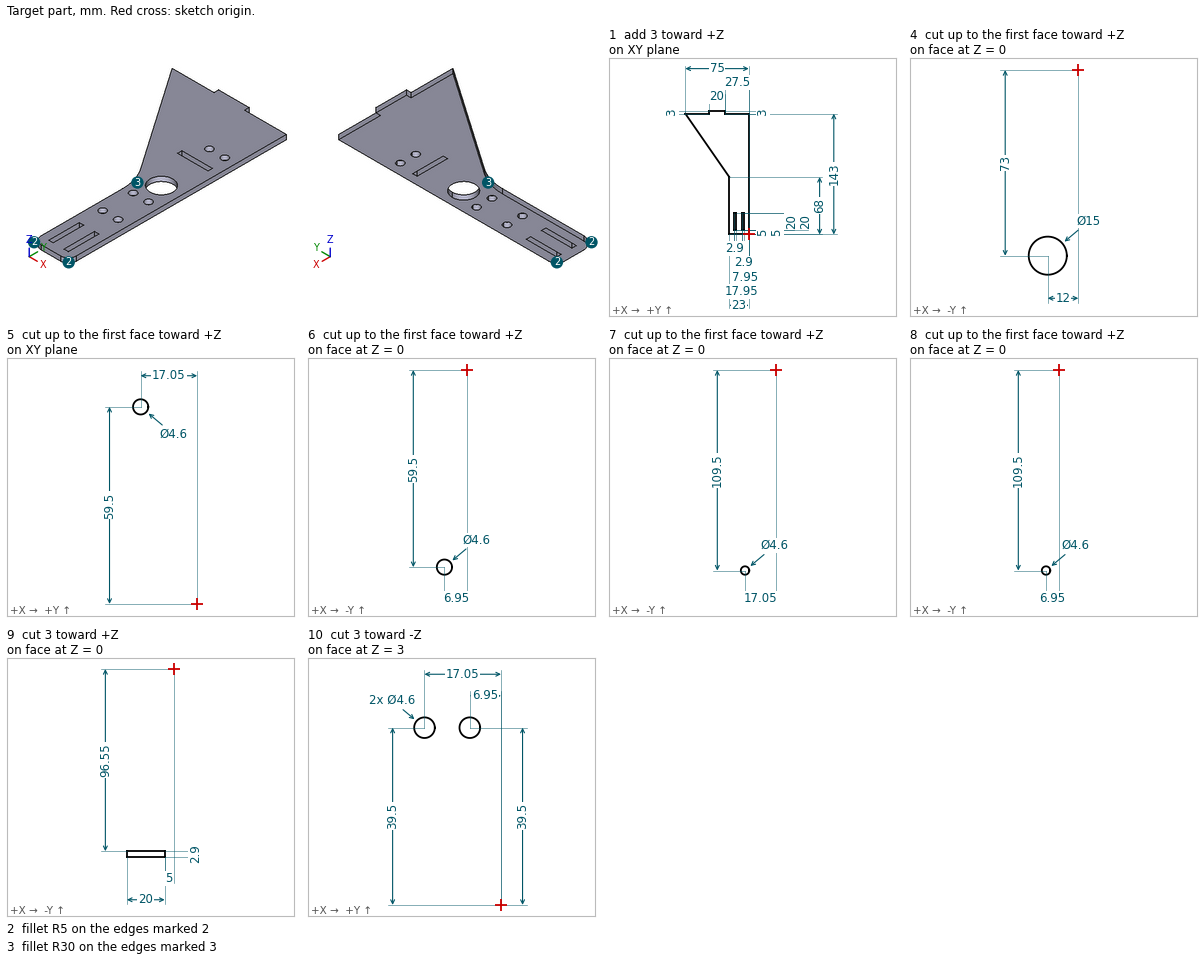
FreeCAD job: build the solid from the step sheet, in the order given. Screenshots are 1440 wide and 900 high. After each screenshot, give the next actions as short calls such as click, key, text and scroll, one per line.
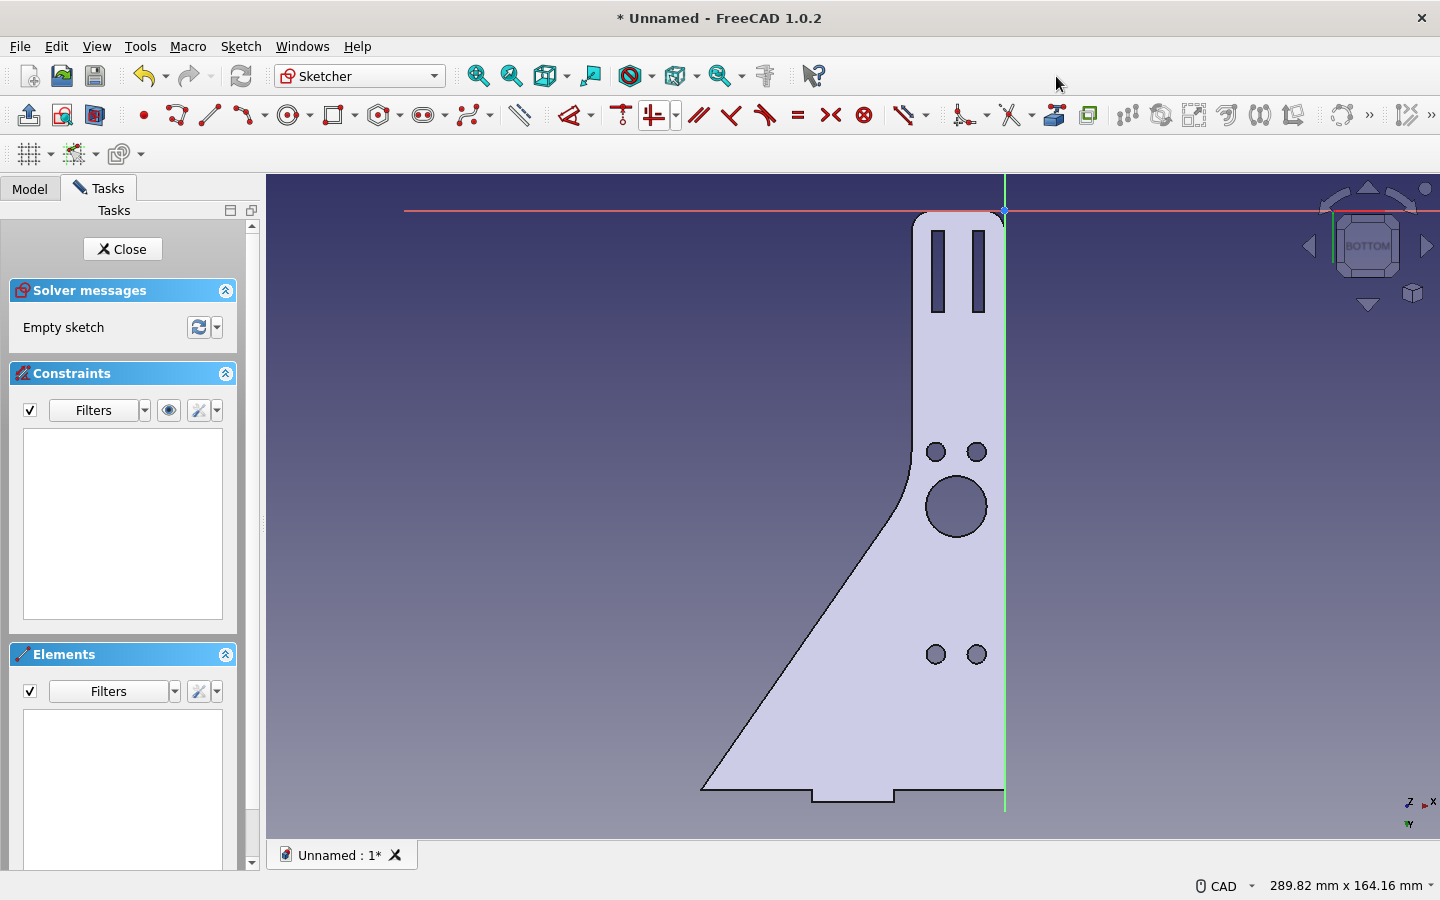
scroll(964, 620, up, 11)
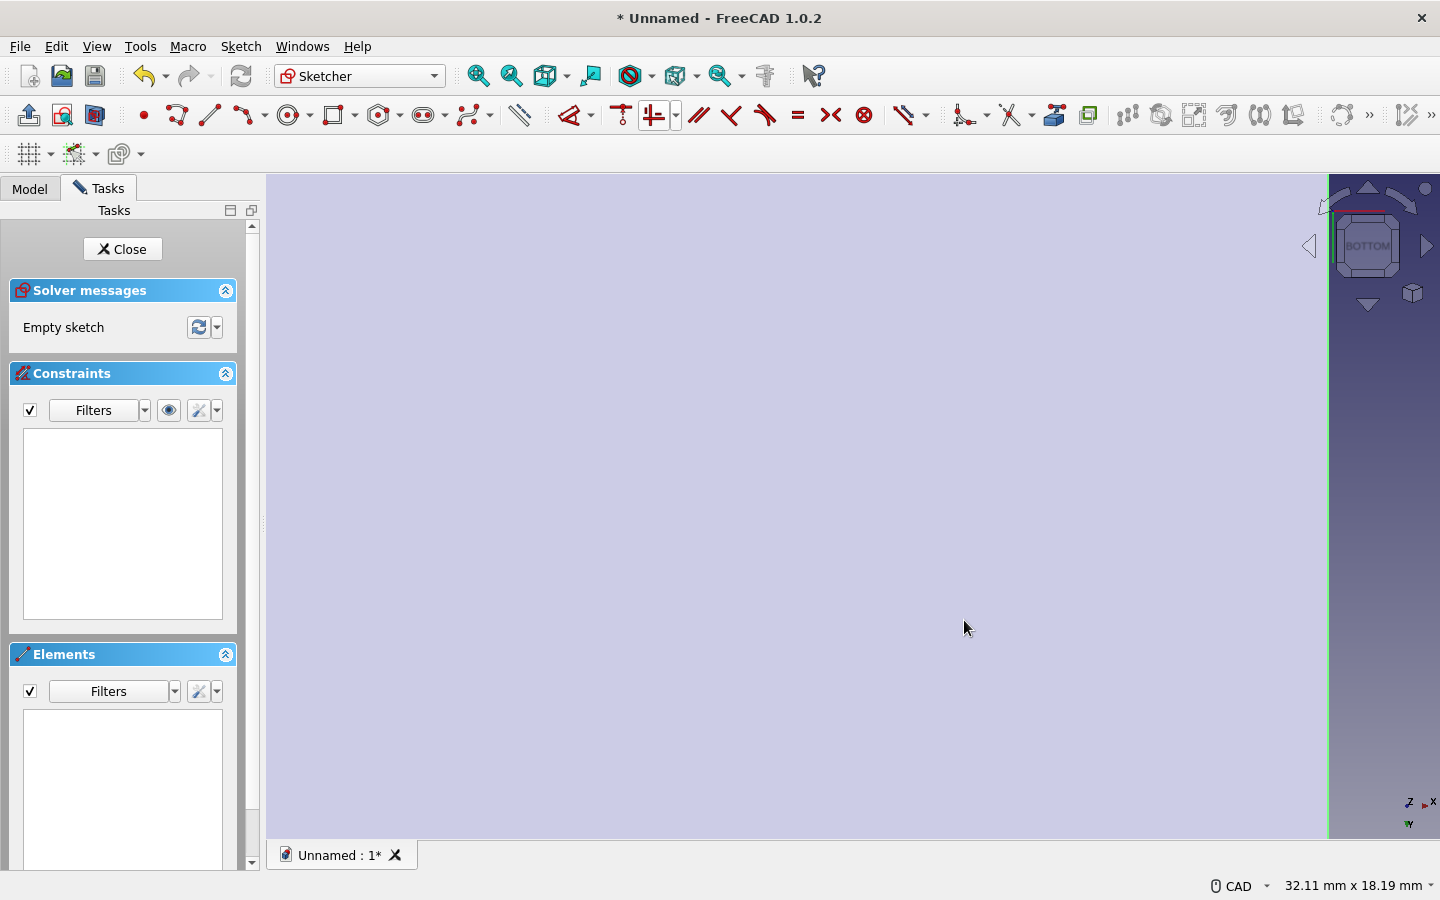
key(g)
key(r)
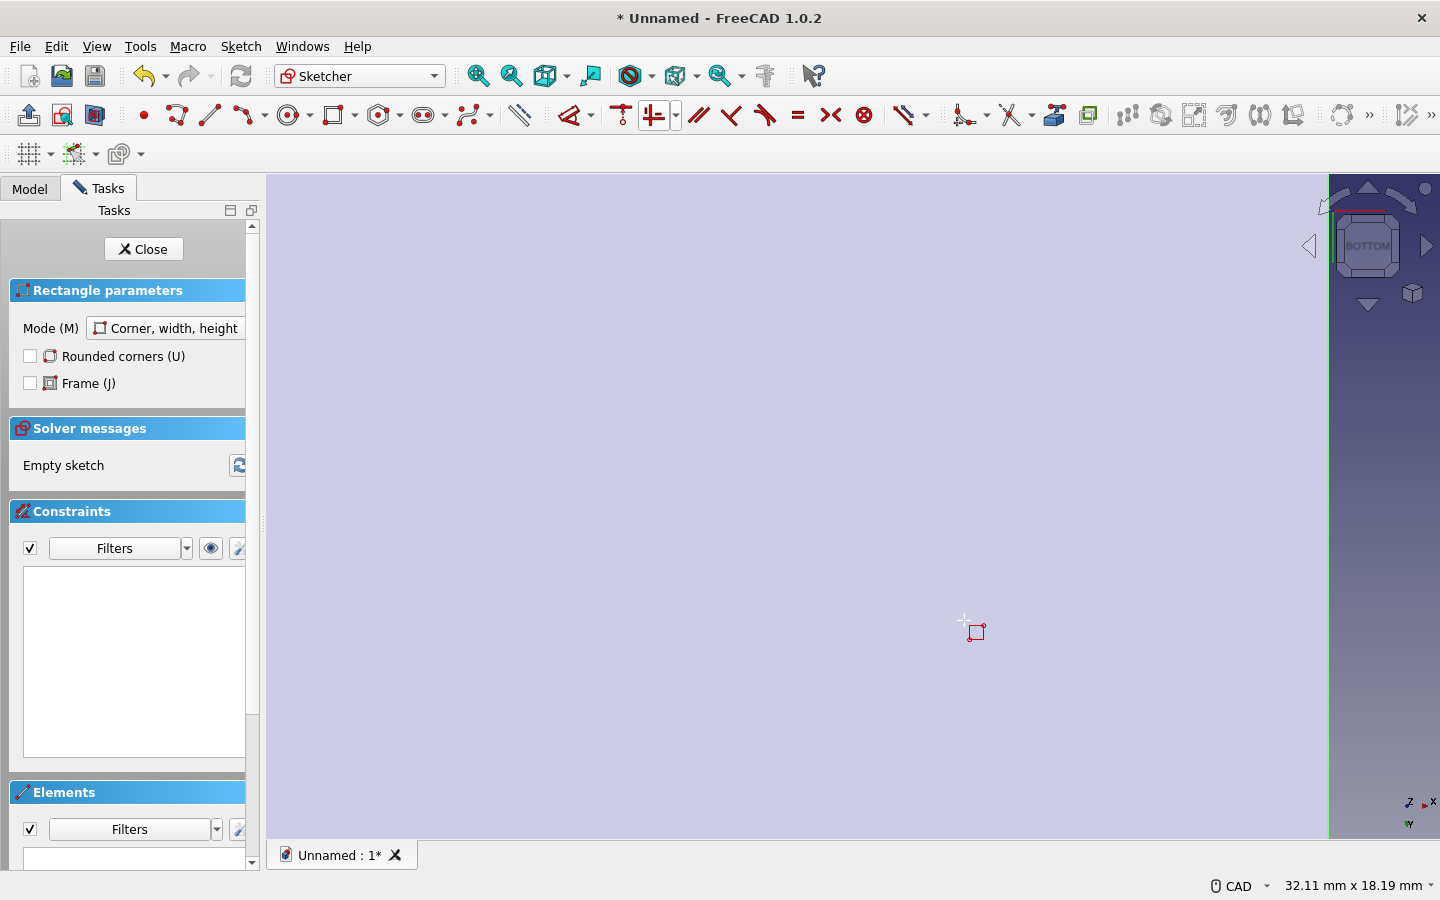
click(414, 451)
move(1146, 557)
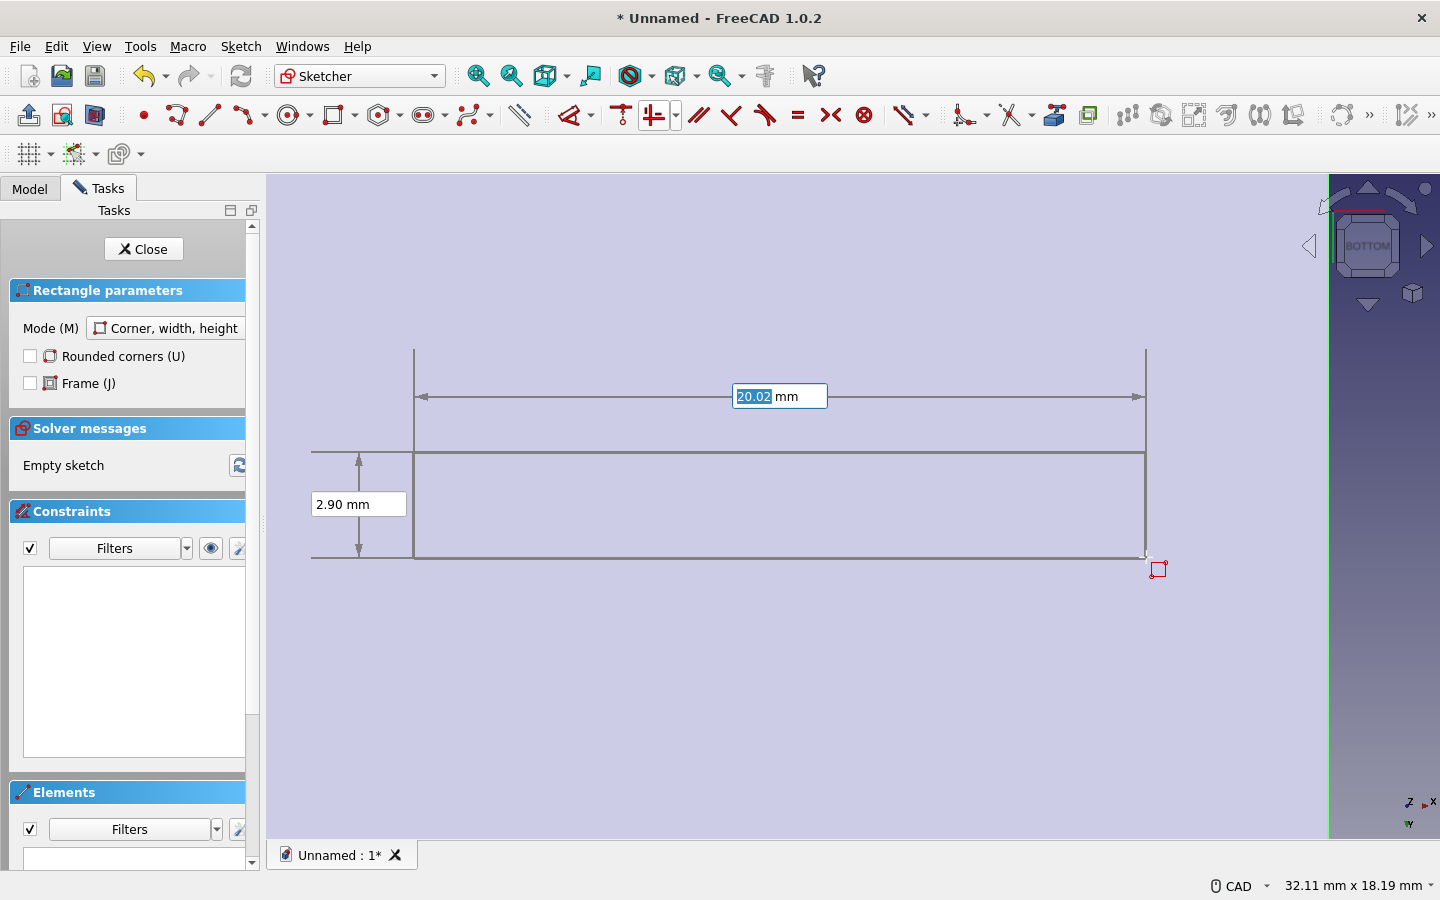
text(20)
key(Tab)
text(2.9)
key(Return)
key(Escape)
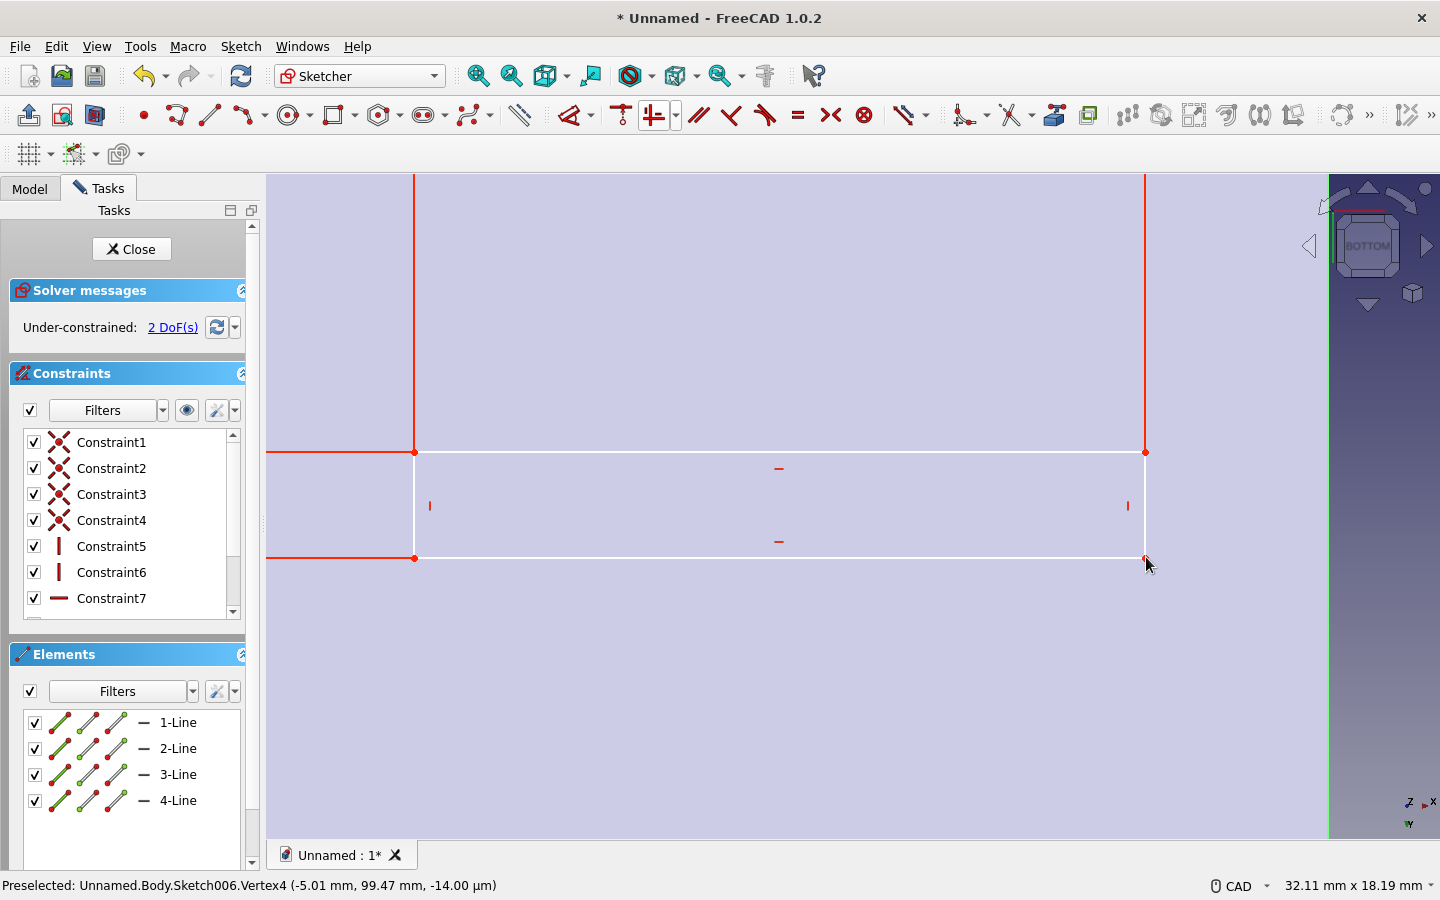
key(d)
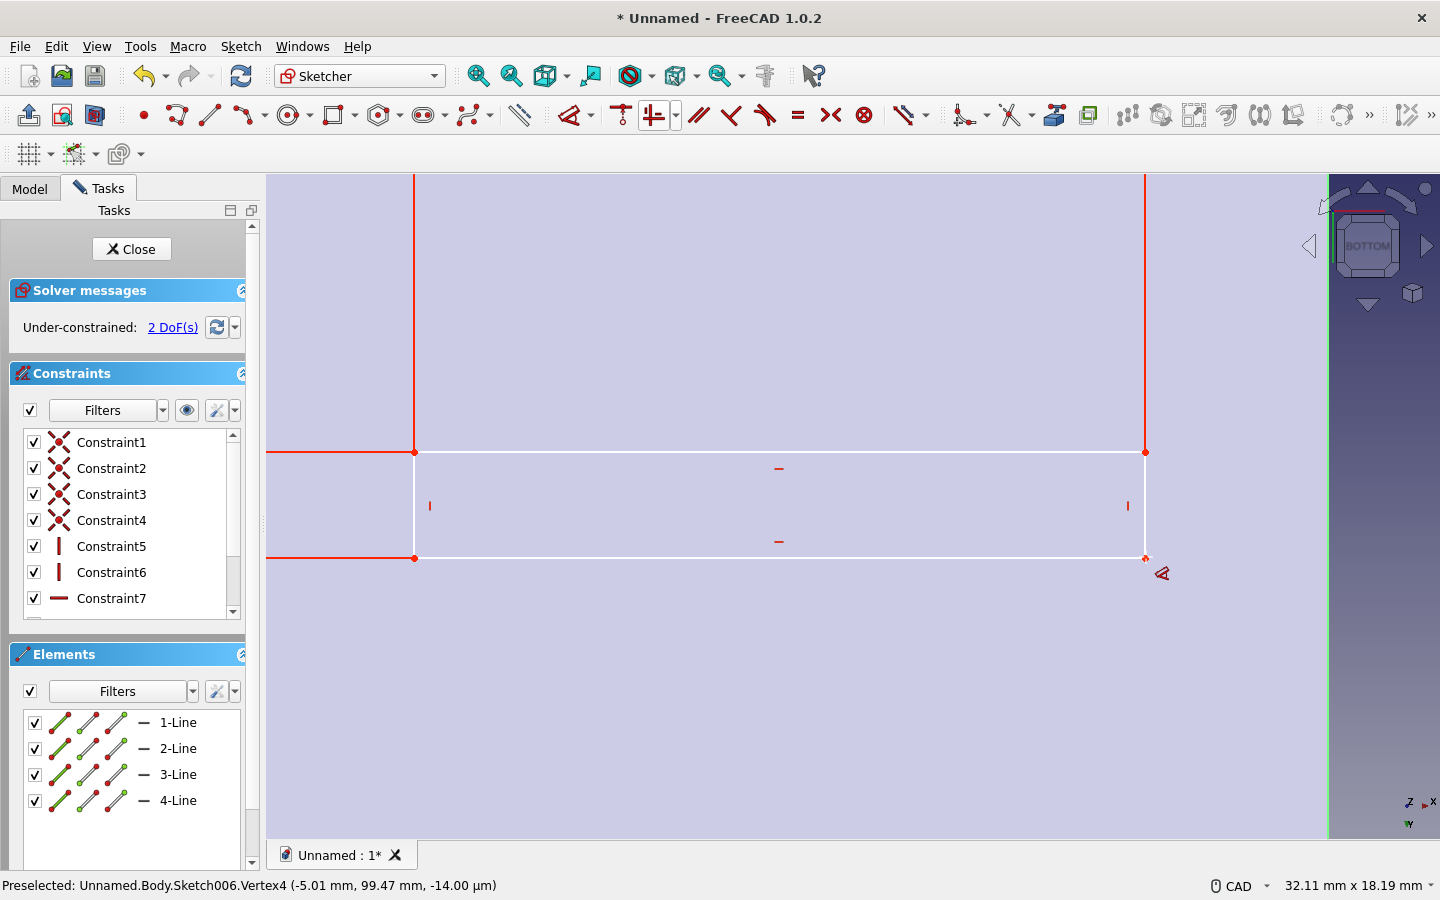
click(1145, 558)
click(1210, 592)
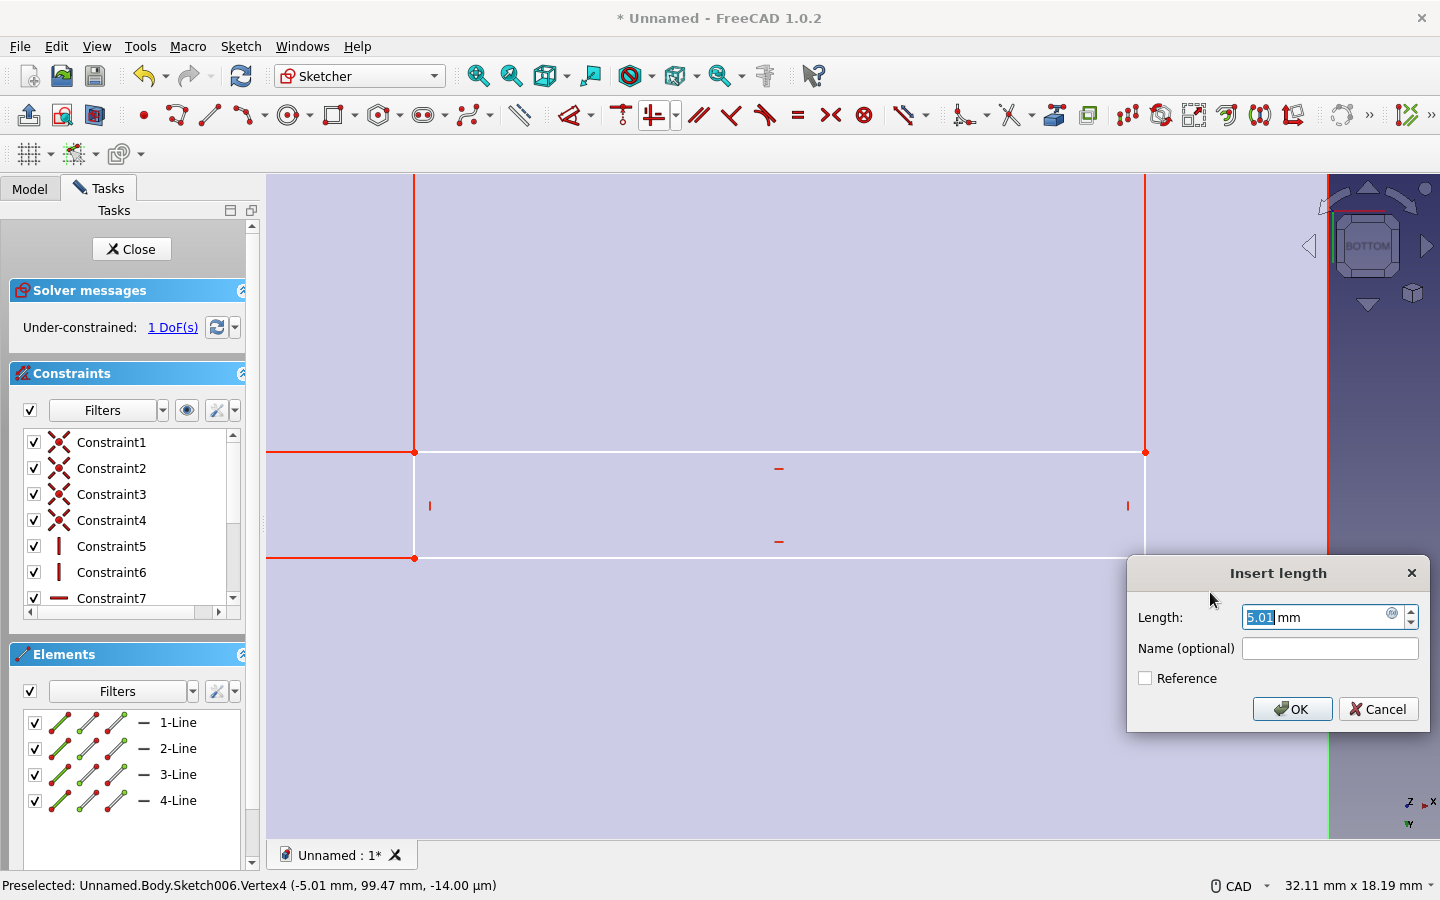
text(5)
key(Return)